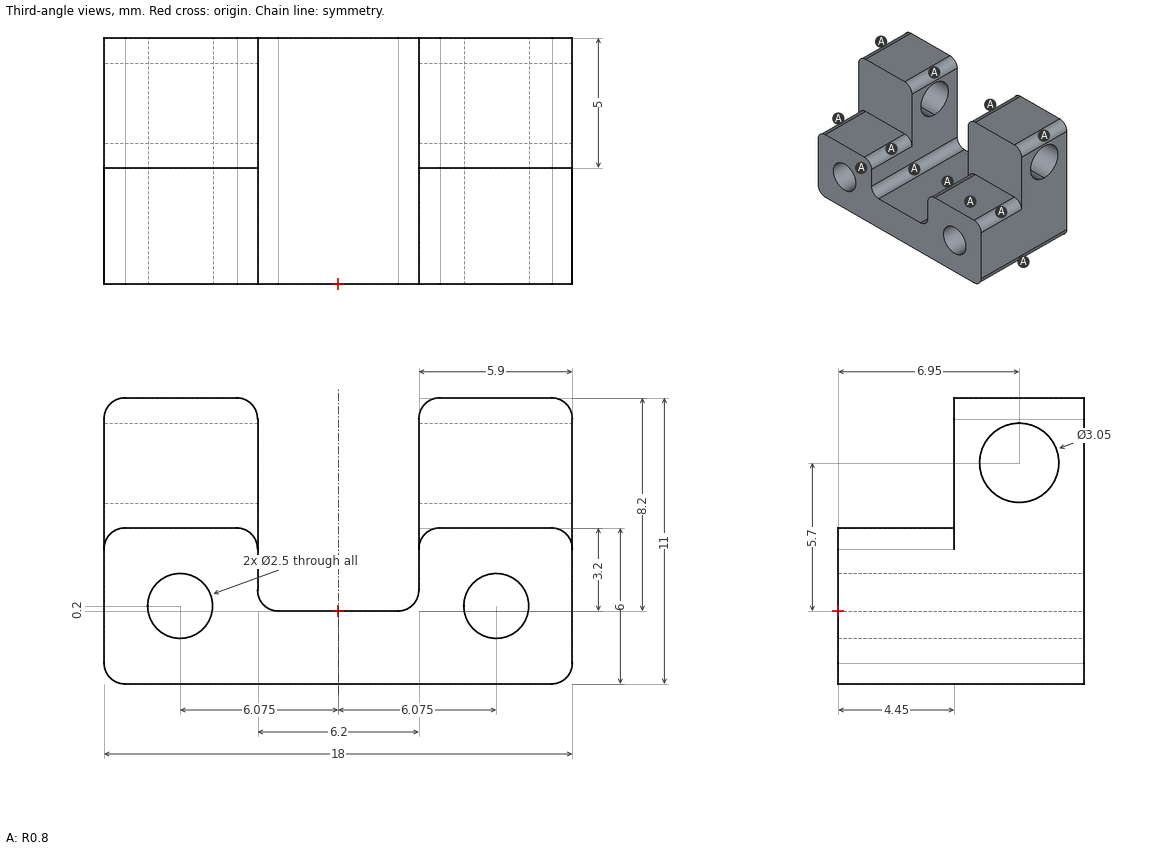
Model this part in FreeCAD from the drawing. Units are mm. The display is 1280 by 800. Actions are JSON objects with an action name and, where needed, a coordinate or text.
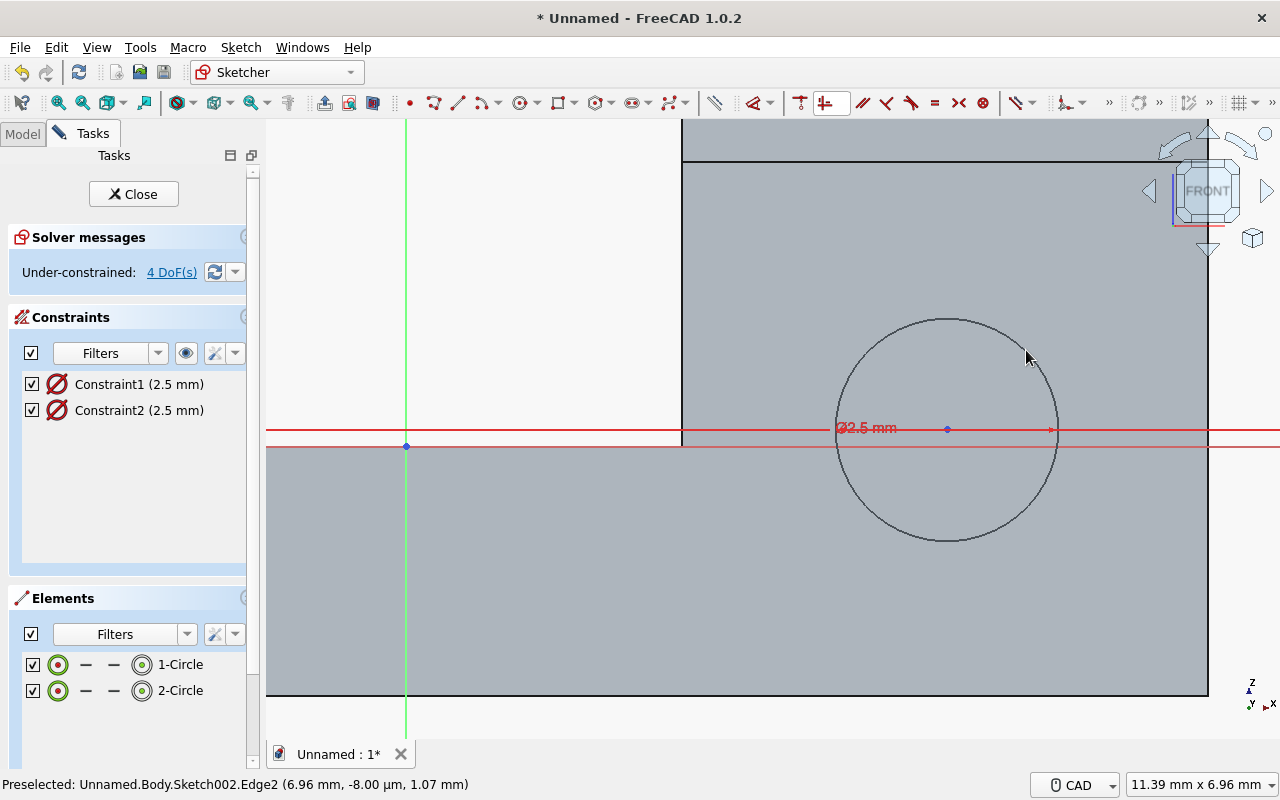
{"action": "scroll", "coordinate": [948, 429], "scroll_direction": "down", "scroll_amount": 4}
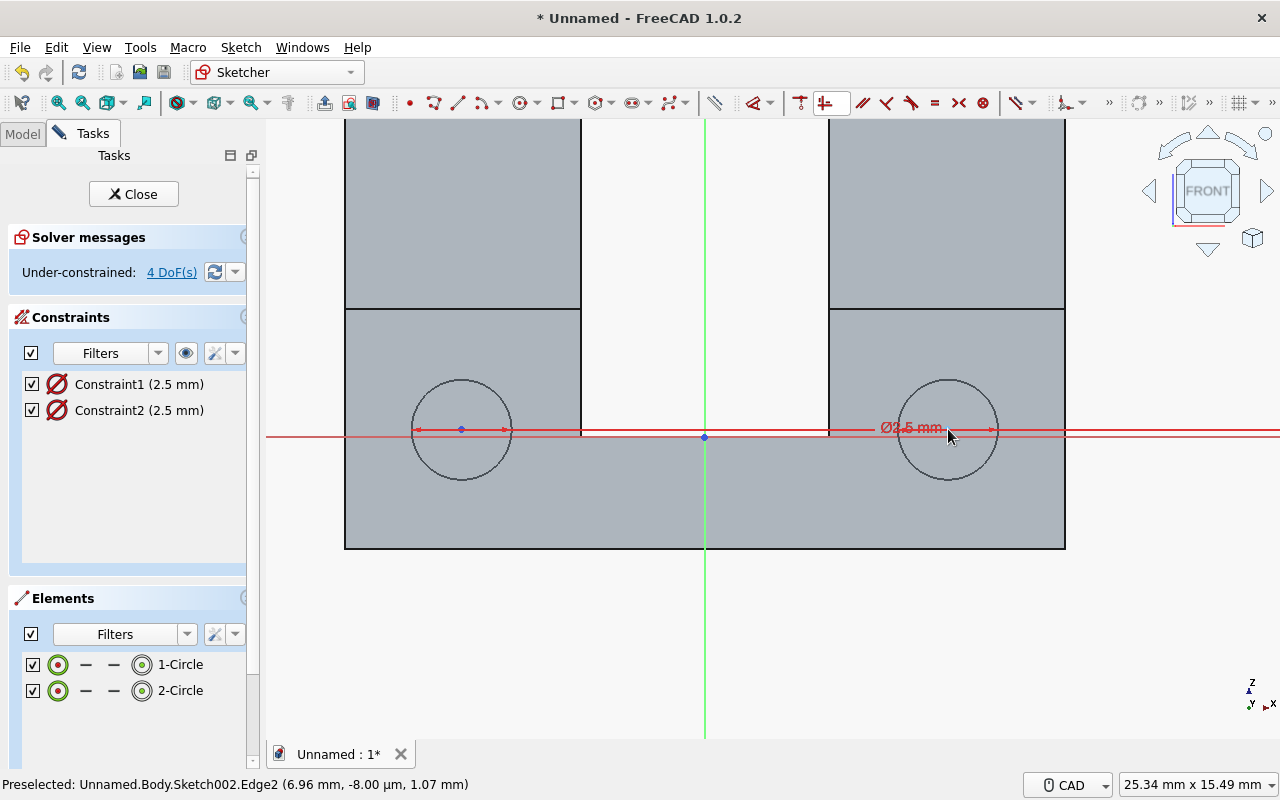
{"action": "left_click", "coordinate": [462, 430]}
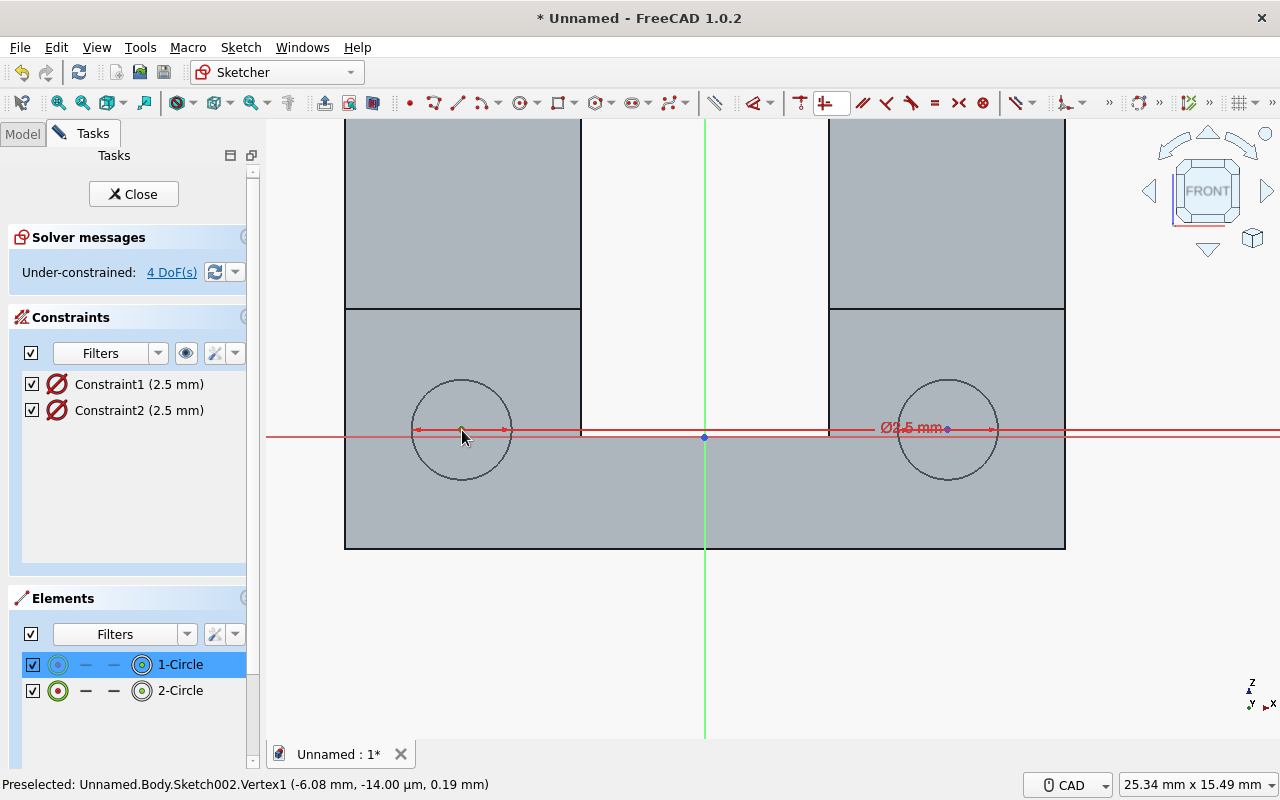
{"action": "left_click", "coordinate": [948, 430]}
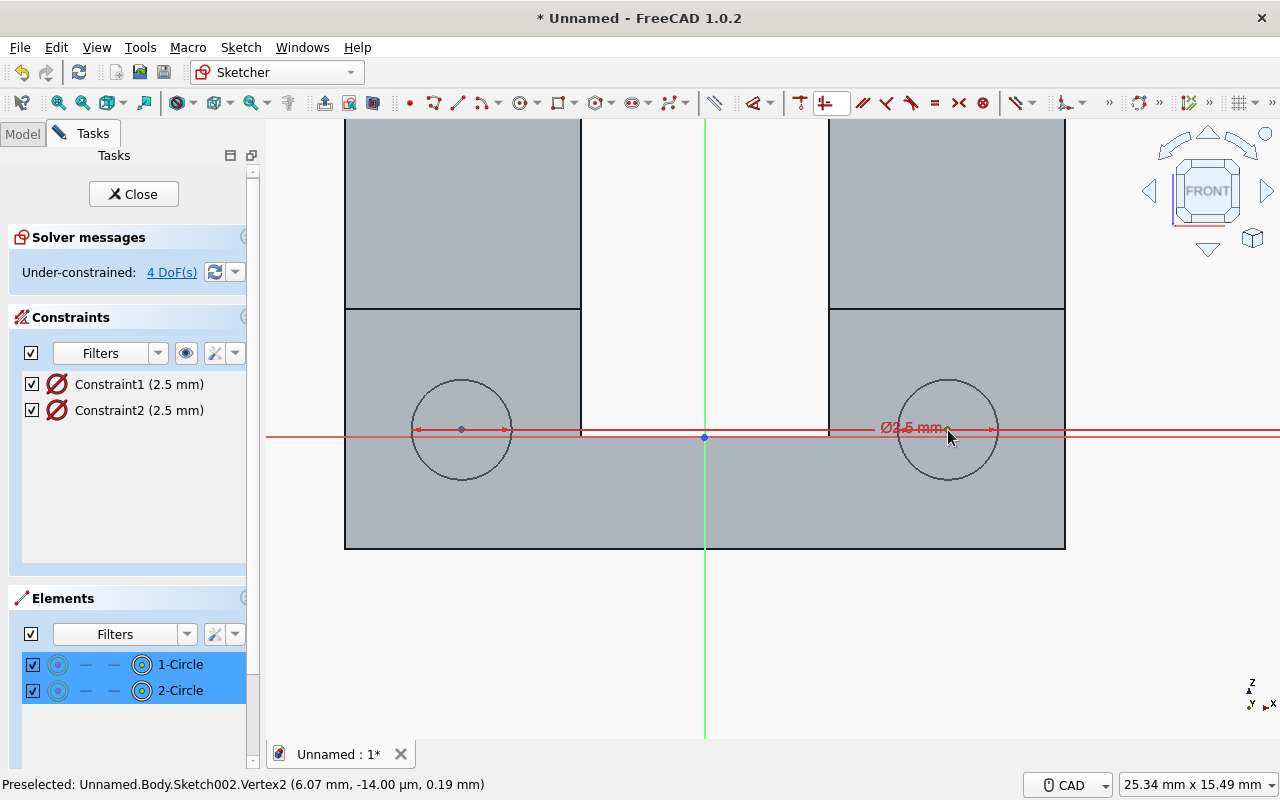
{"action": "key", "text": "h"}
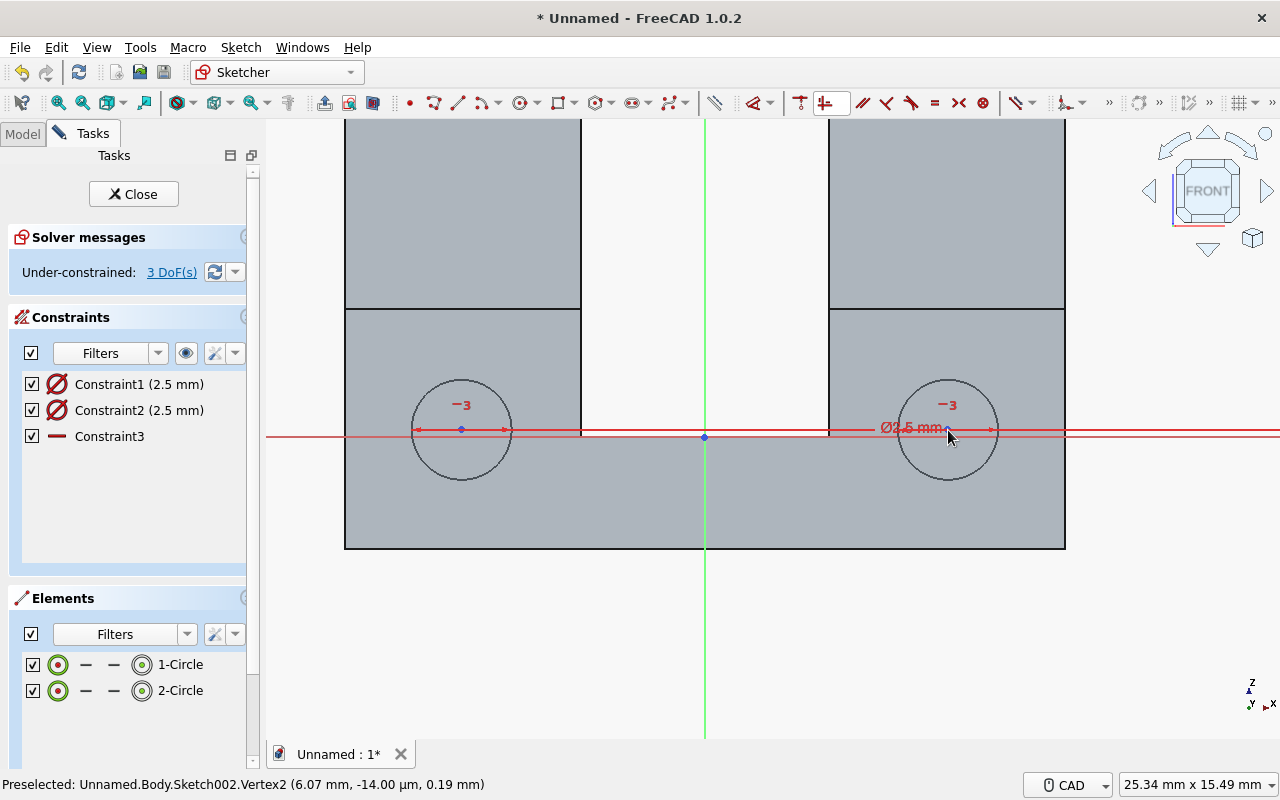
{"action": "left_click", "coordinate": [754, 104]}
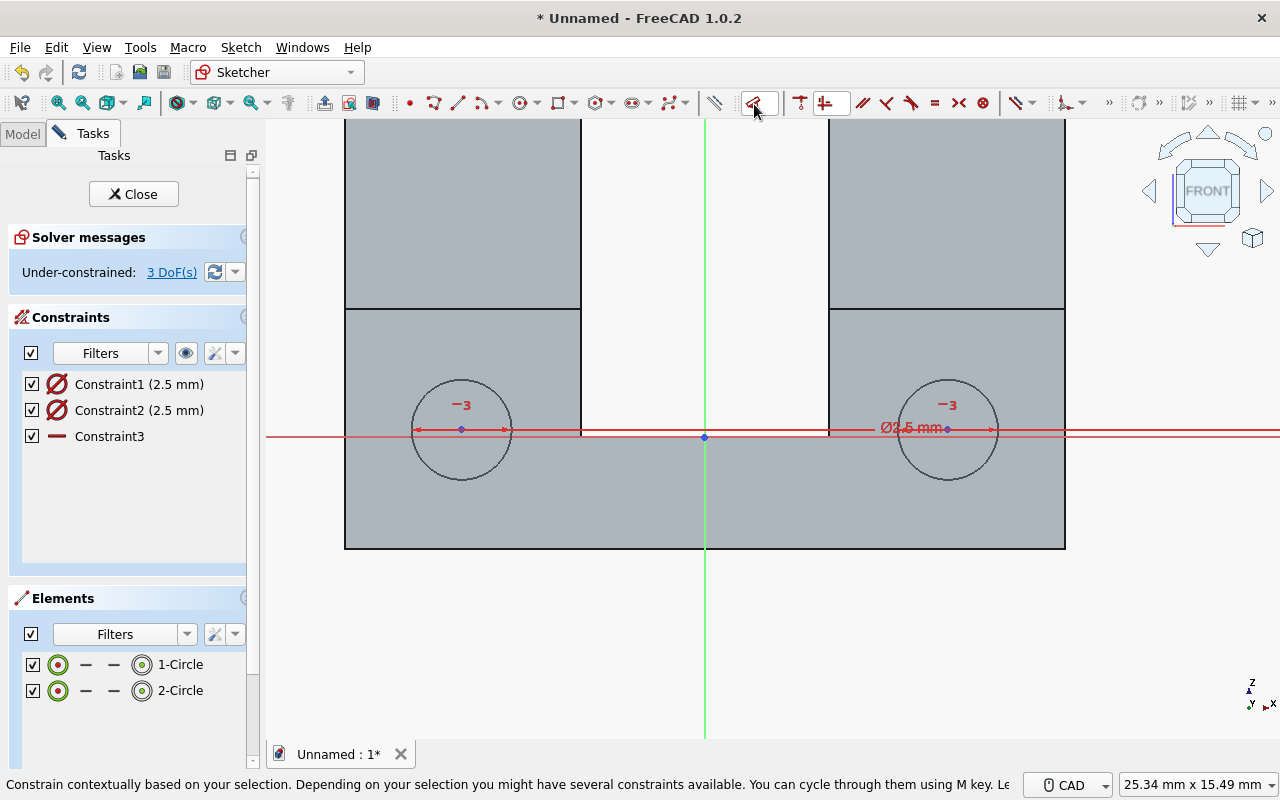
{"action": "scroll", "coordinate": [462, 430], "scroll_direction": "up", "scroll_amount": 9}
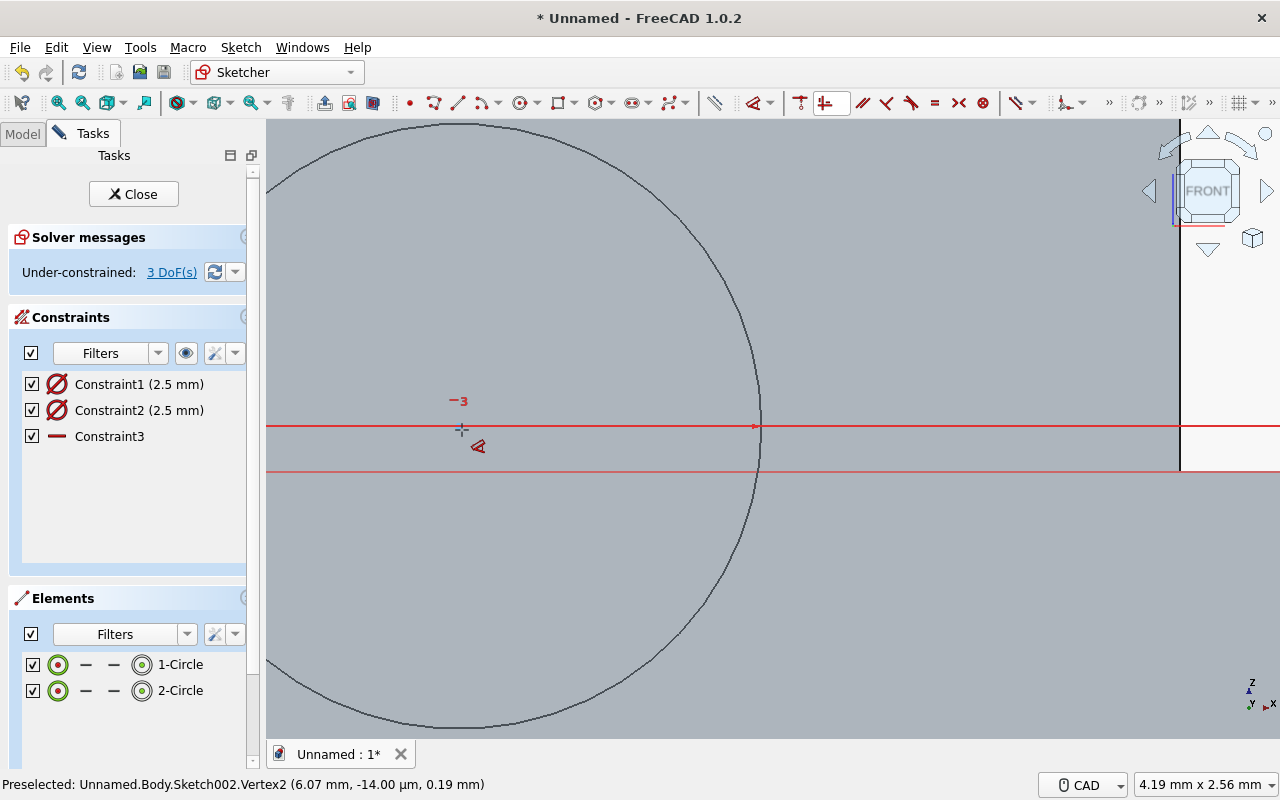
{"action": "left_click", "coordinate": [459, 426]}
{"action": "left_click", "coordinate": [425, 449]}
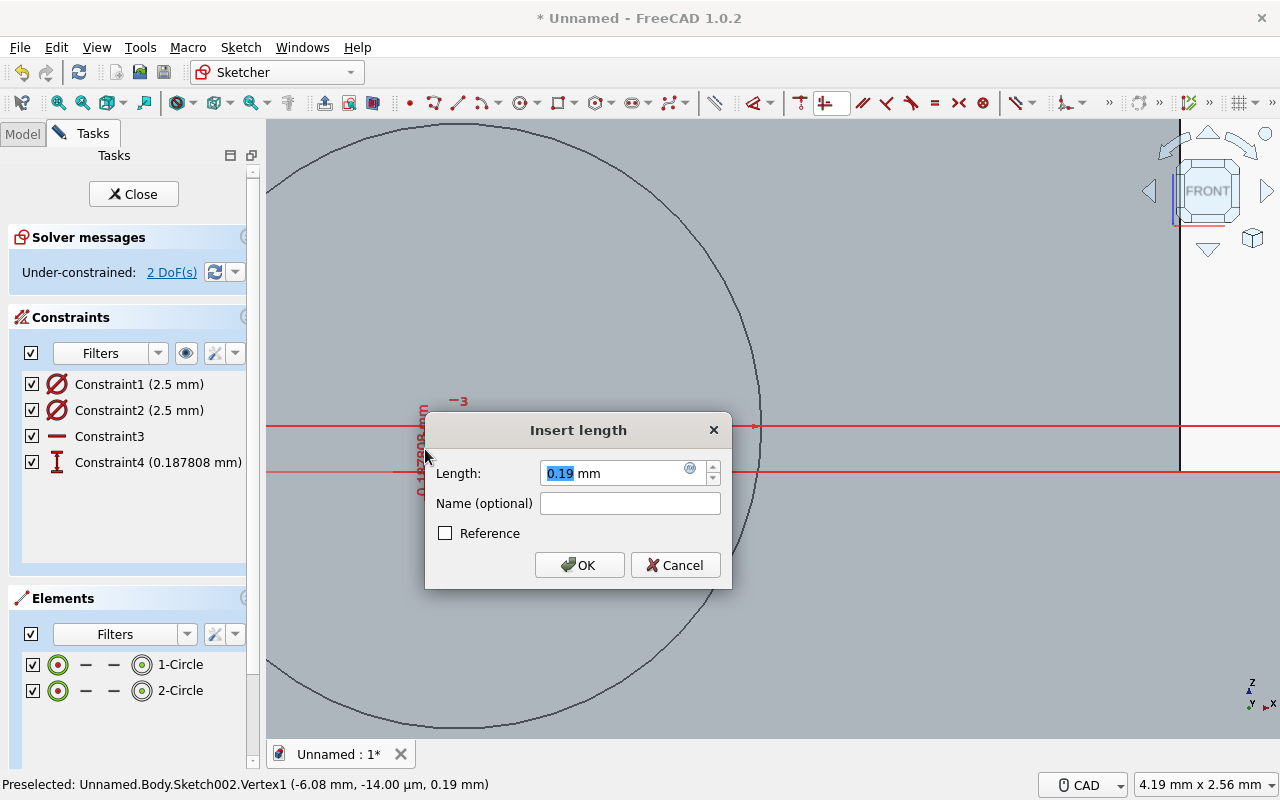
{"action": "type", "text": "0.2"}
{"action": "key", "text": "Return"}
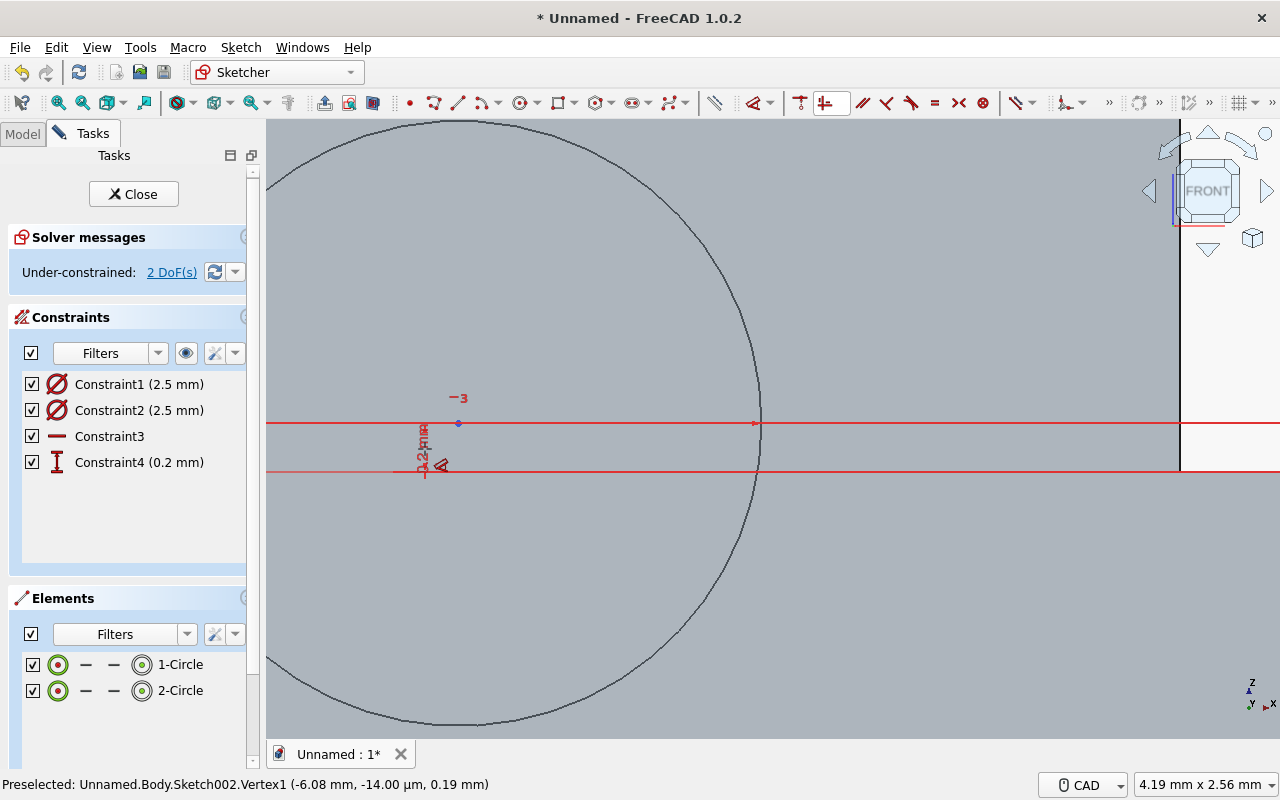
{"action": "scroll", "coordinate": [462, 430], "scroll_direction": "down", "scroll_amount": 9}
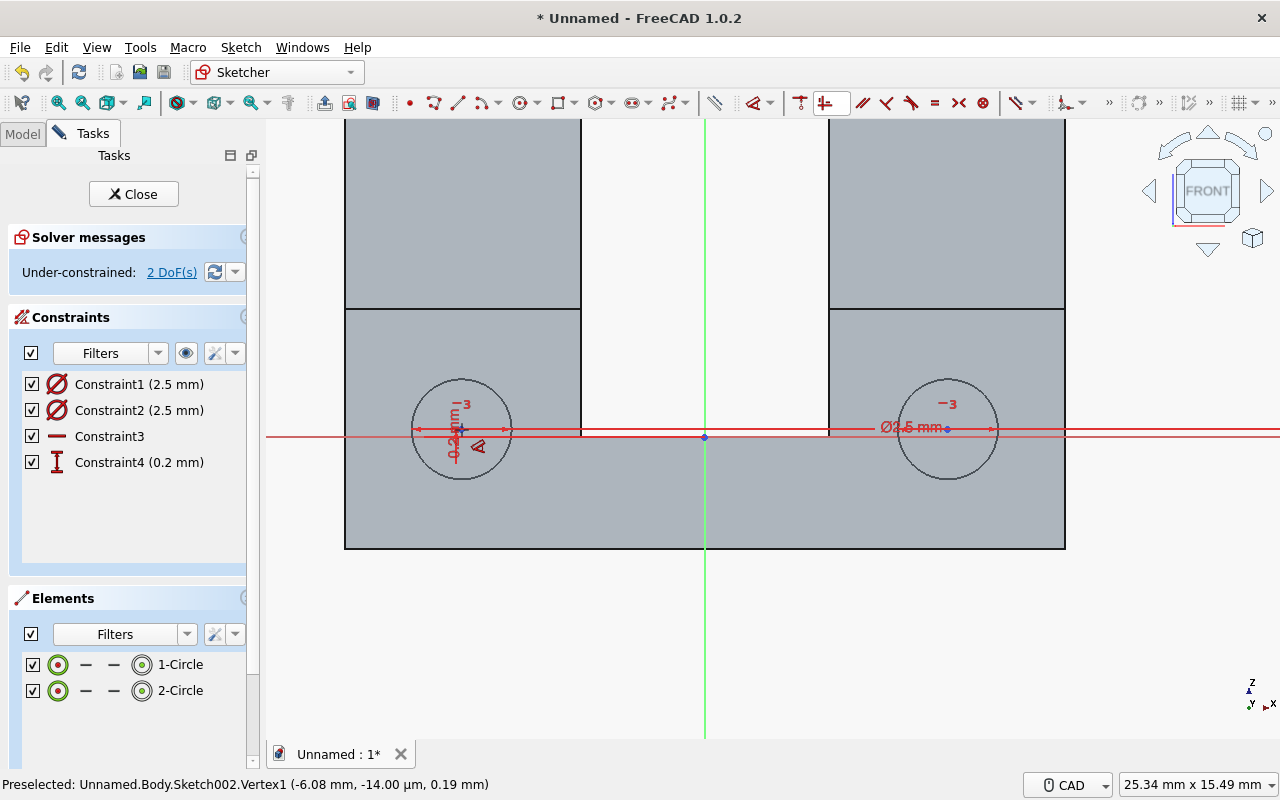
{"action": "left_click", "coordinate": [462, 429]}
{"action": "left_click", "coordinate": [583, 471]}